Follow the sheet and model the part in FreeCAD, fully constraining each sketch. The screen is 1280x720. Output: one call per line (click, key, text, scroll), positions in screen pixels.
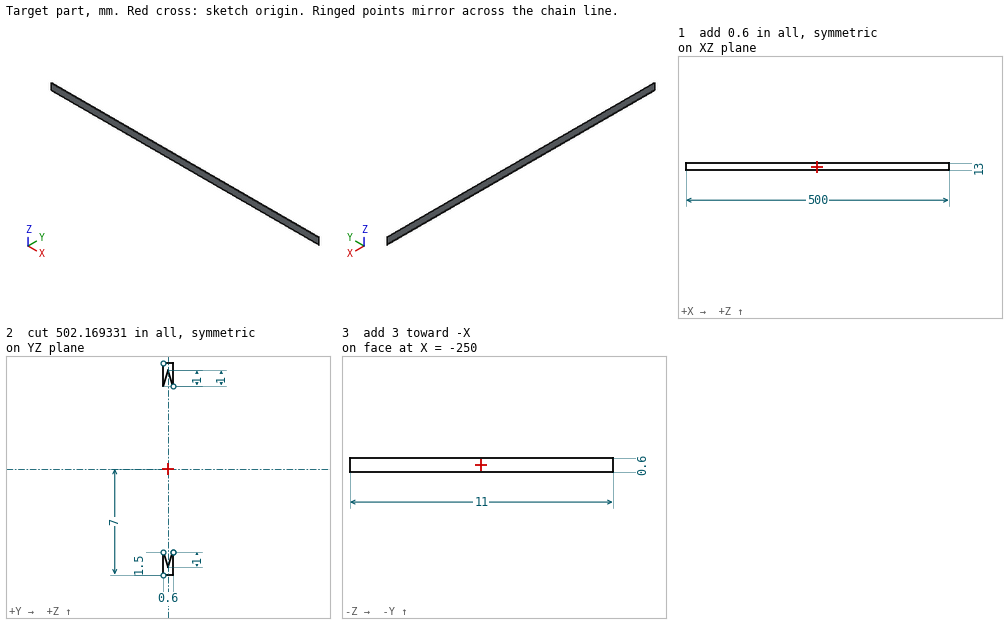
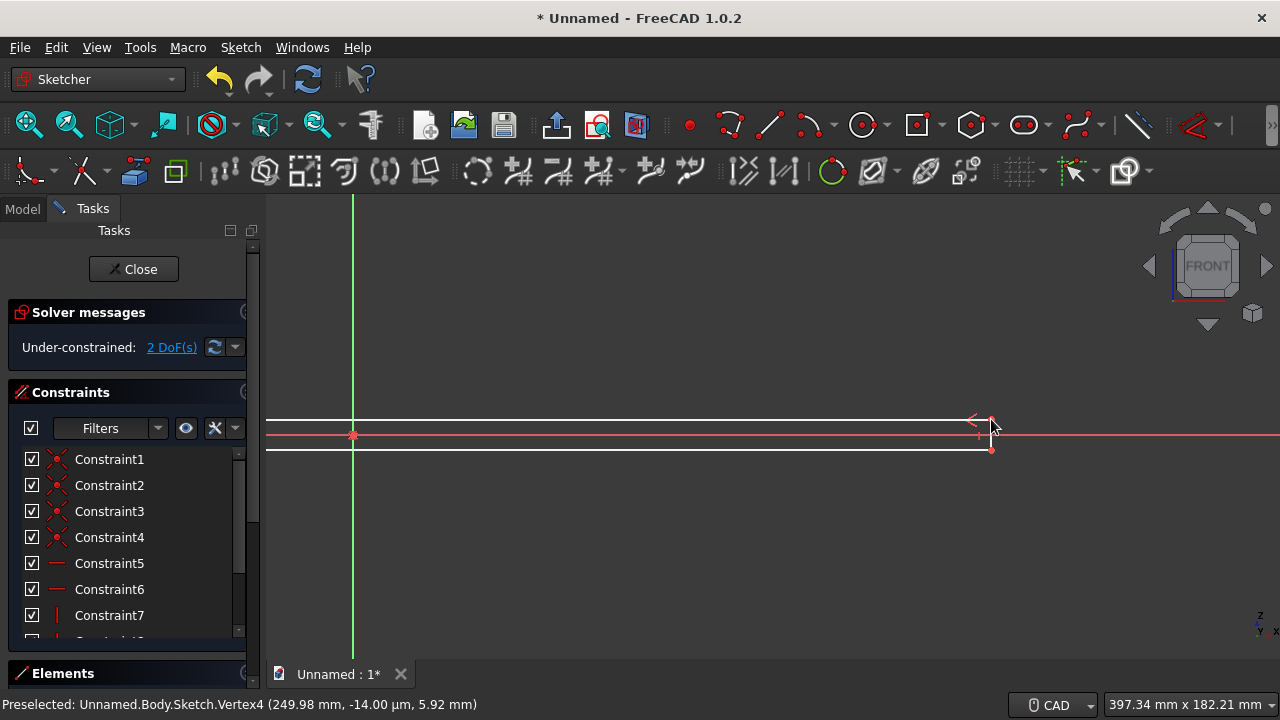
click(1194, 126)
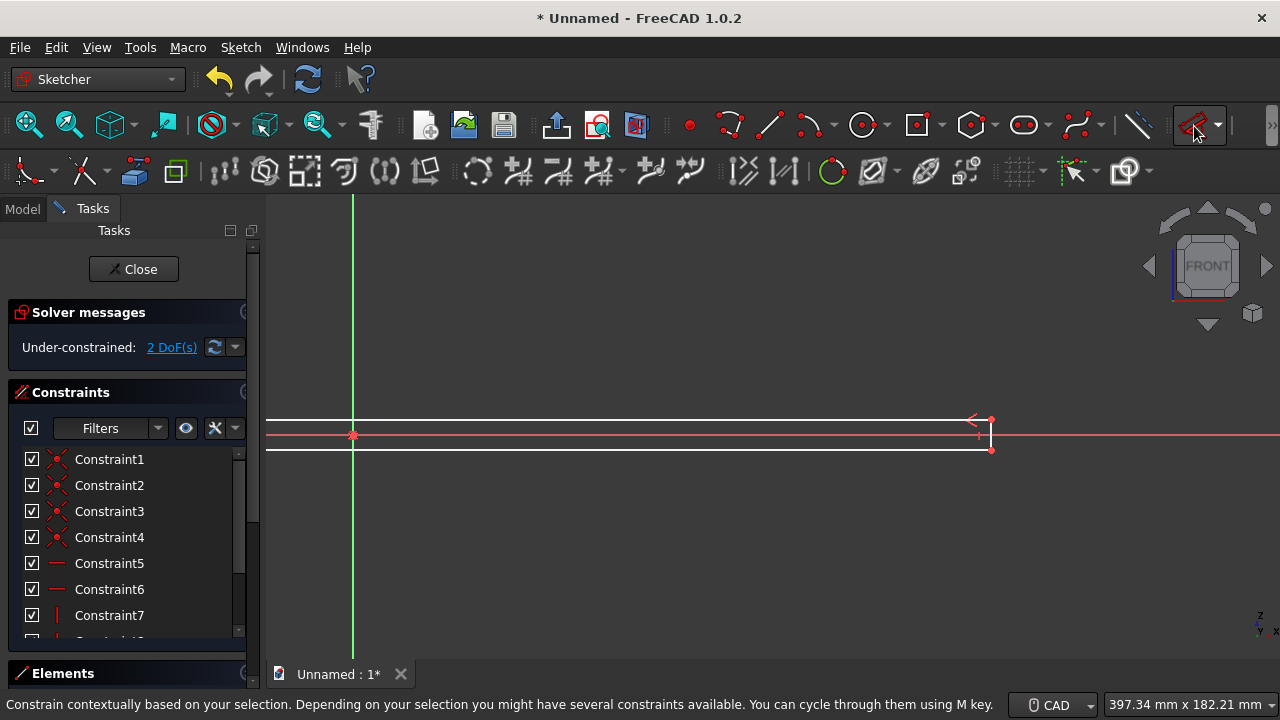
click(991, 438)
click(1025, 428)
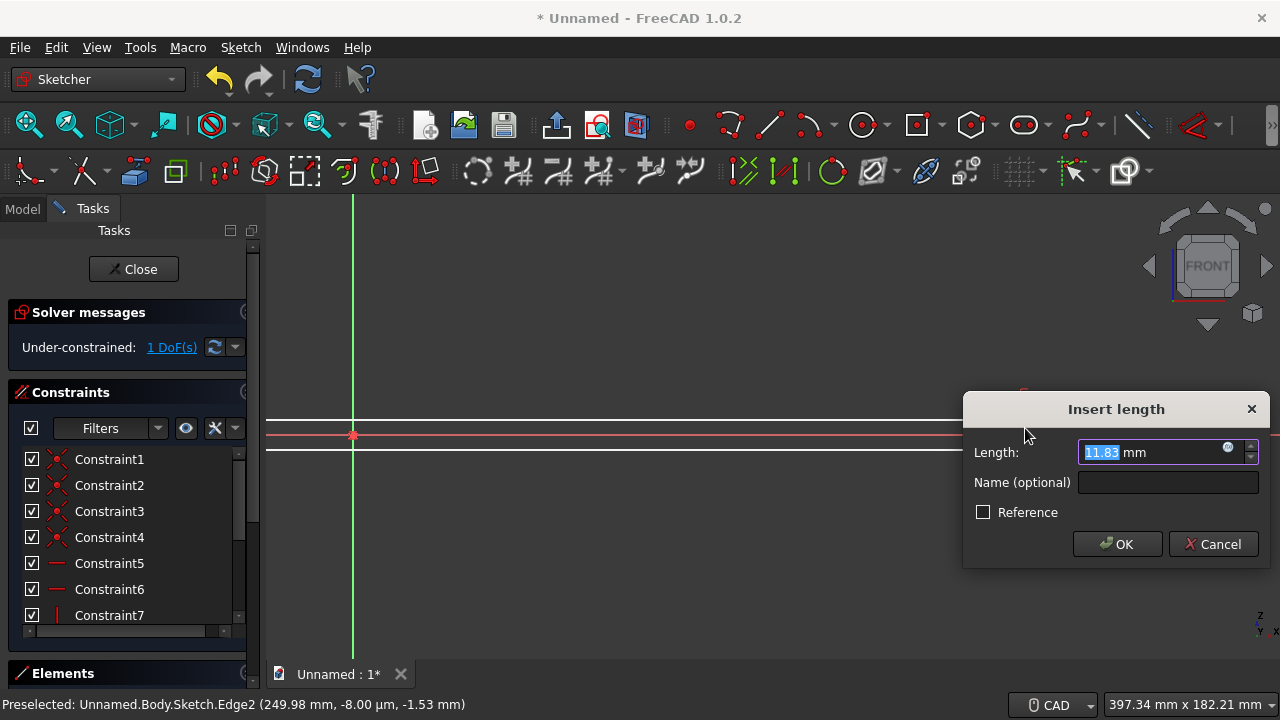
text(13)
key(Return)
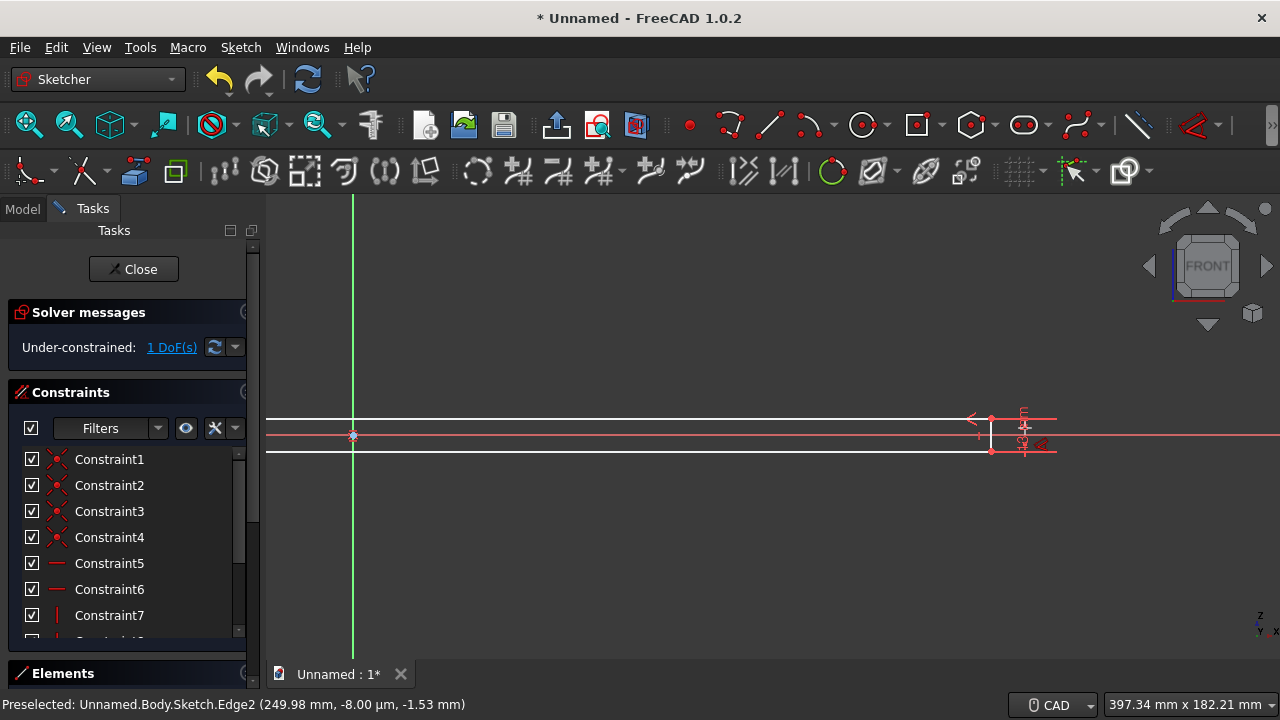
click(608, 452)
click(642, 486)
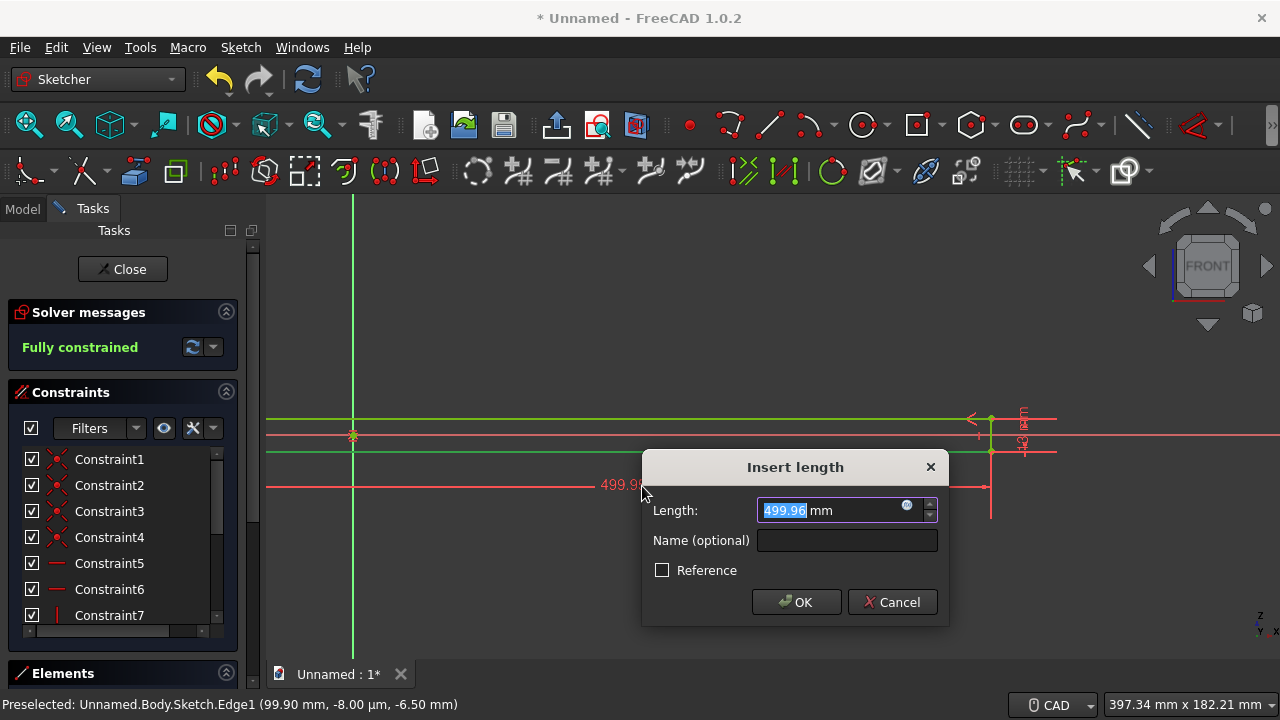
text(500)
key(Return)
key(Escape)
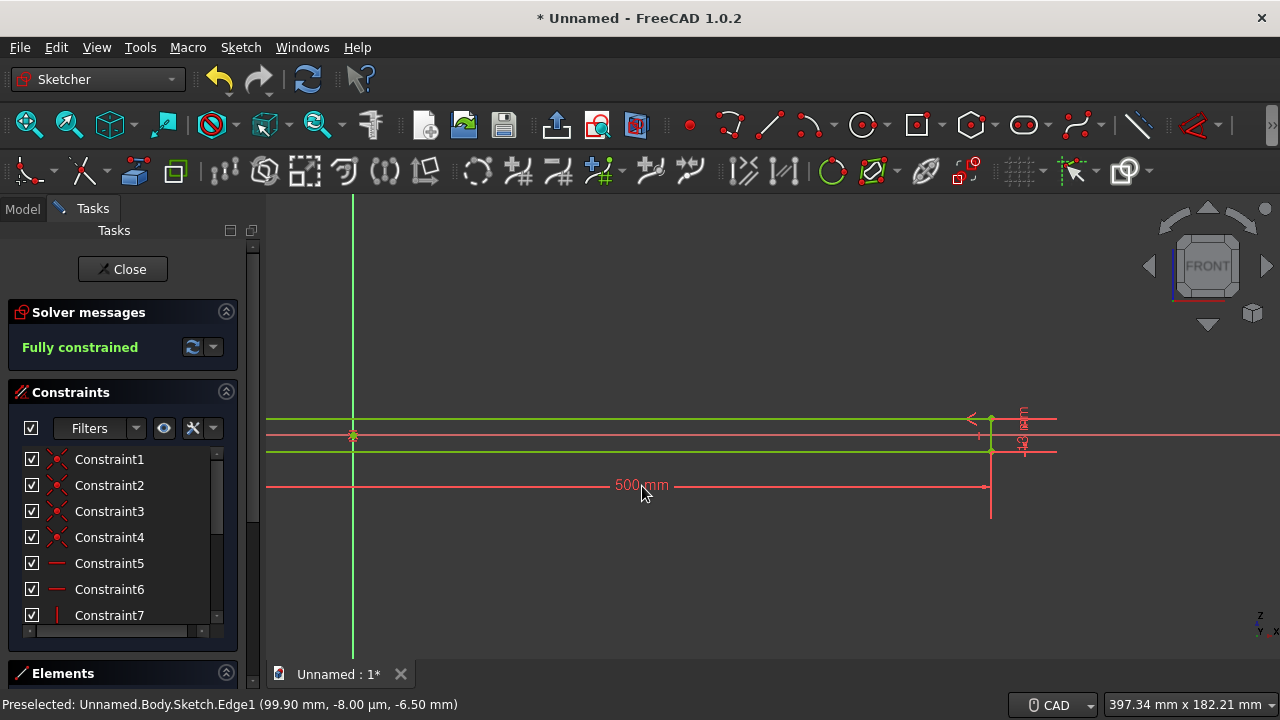
click(123, 269)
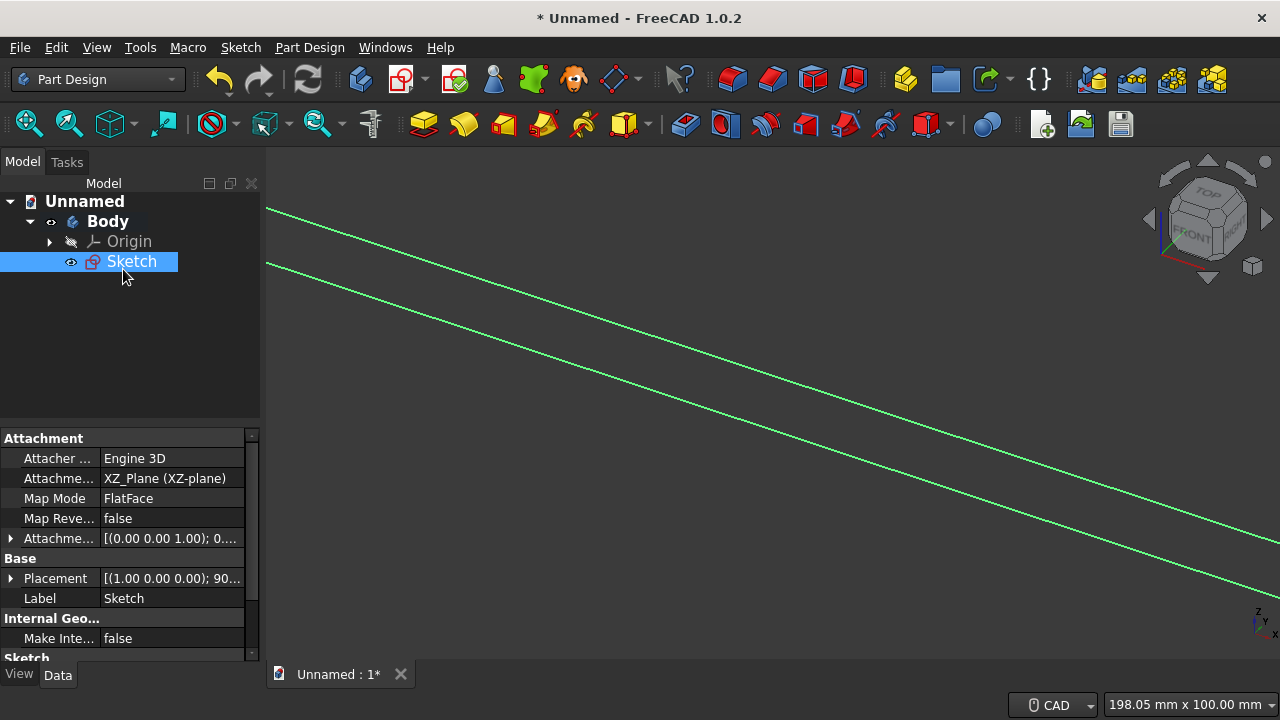
click(424, 124)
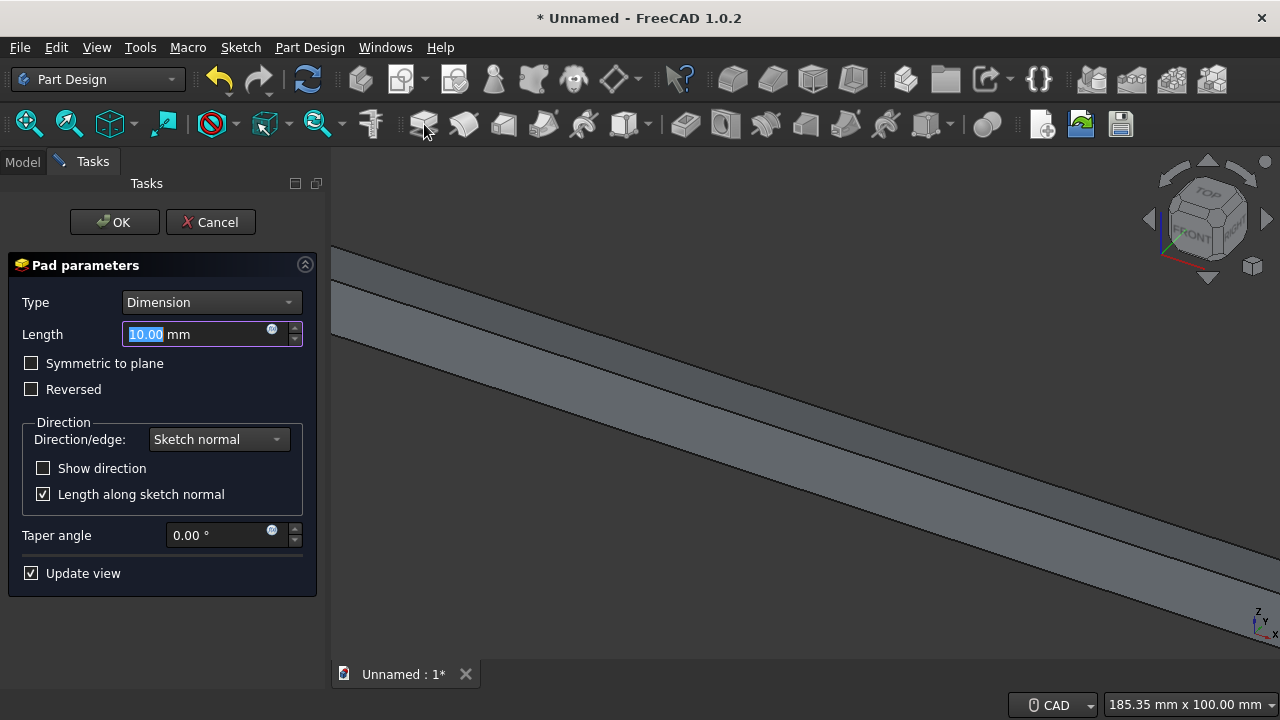
text(0.6)
key(Tab)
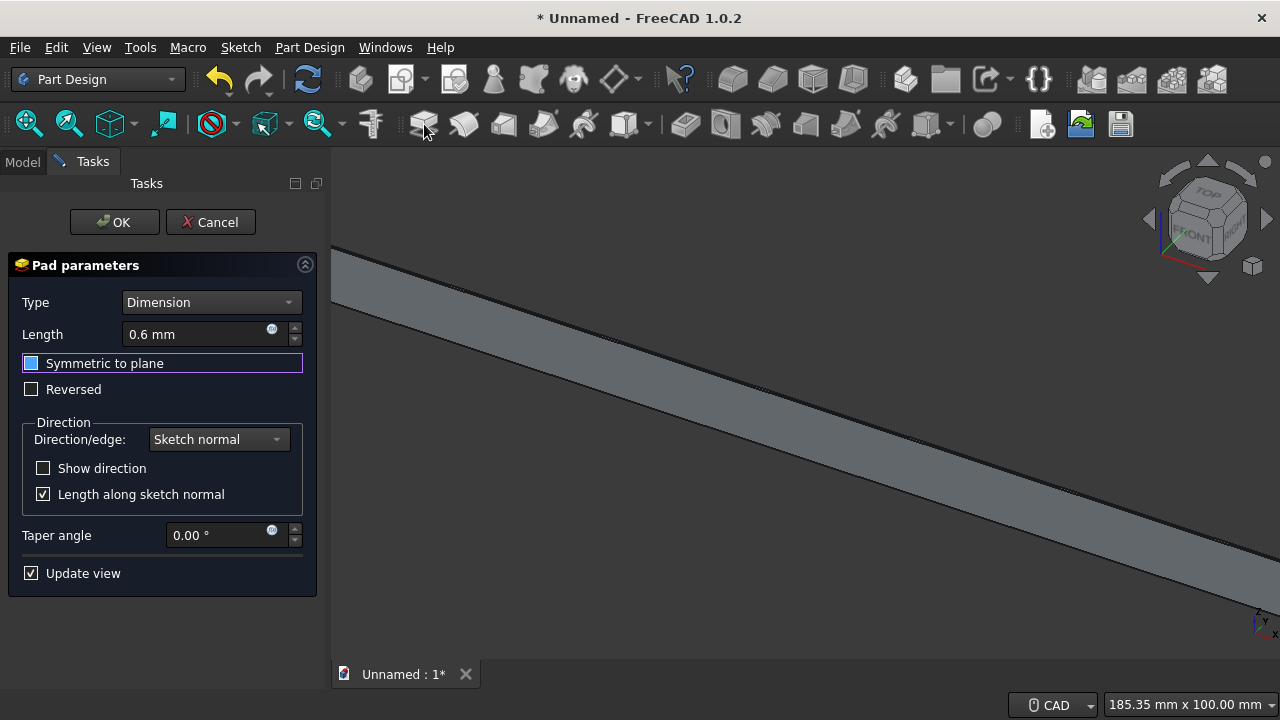
click(30, 363)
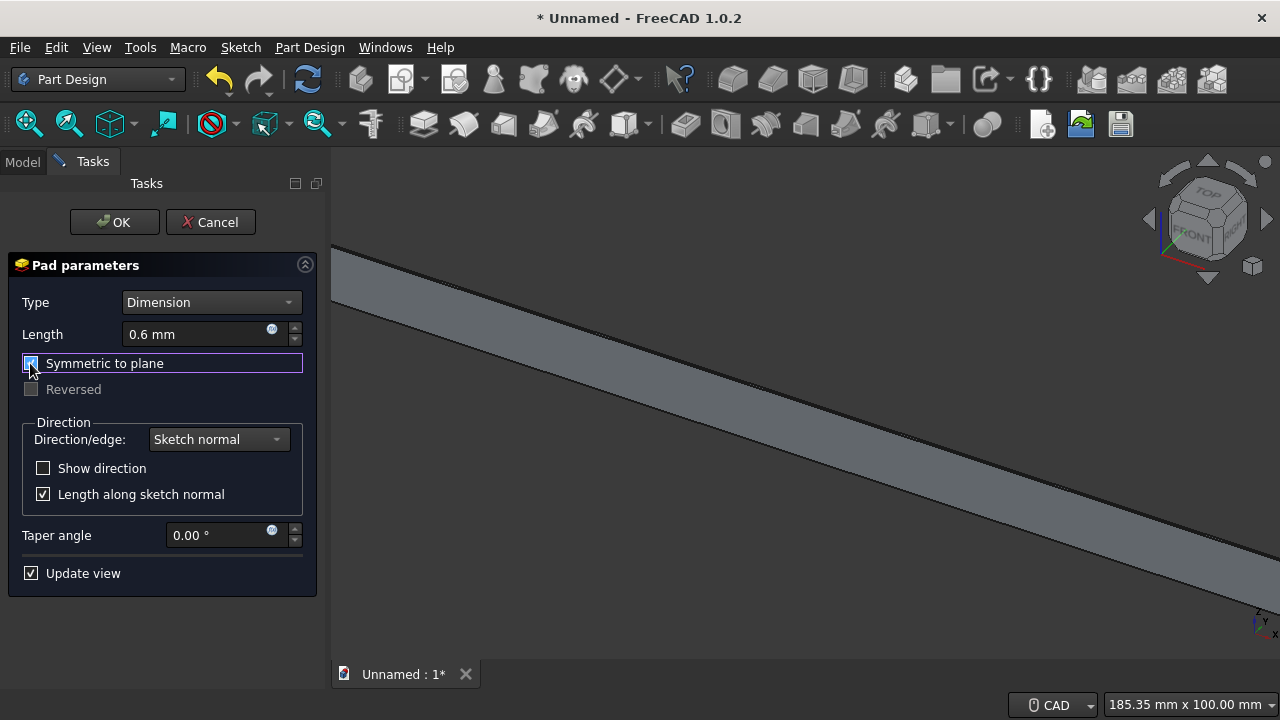
click(115, 222)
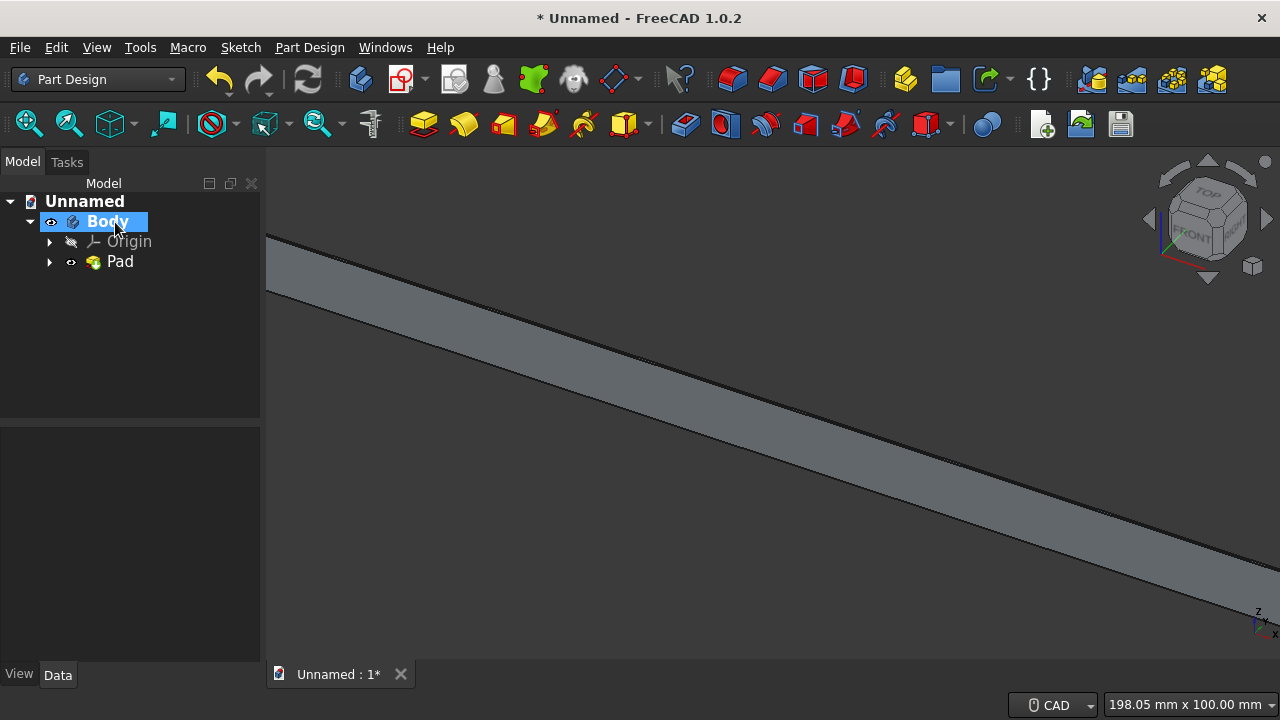
key(v)
key(f)